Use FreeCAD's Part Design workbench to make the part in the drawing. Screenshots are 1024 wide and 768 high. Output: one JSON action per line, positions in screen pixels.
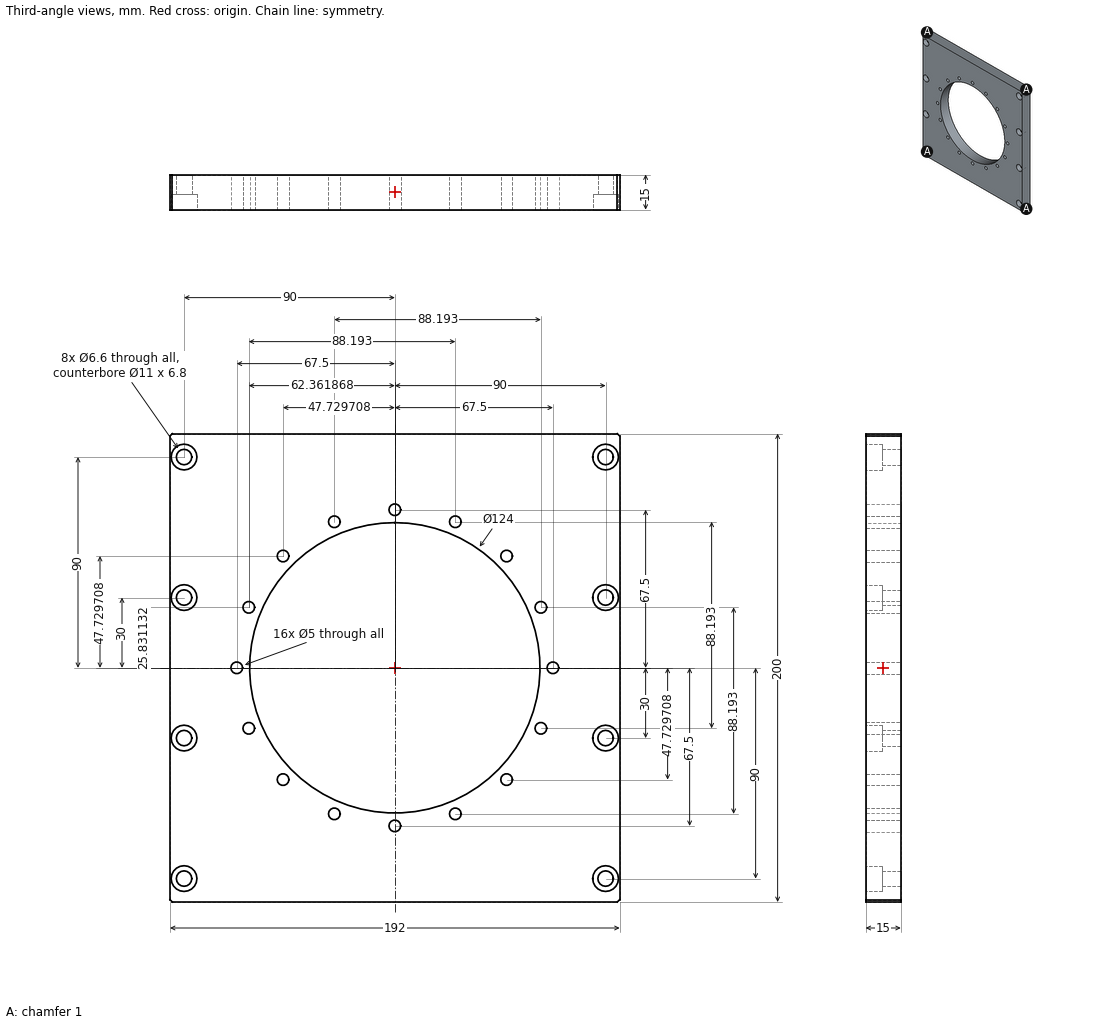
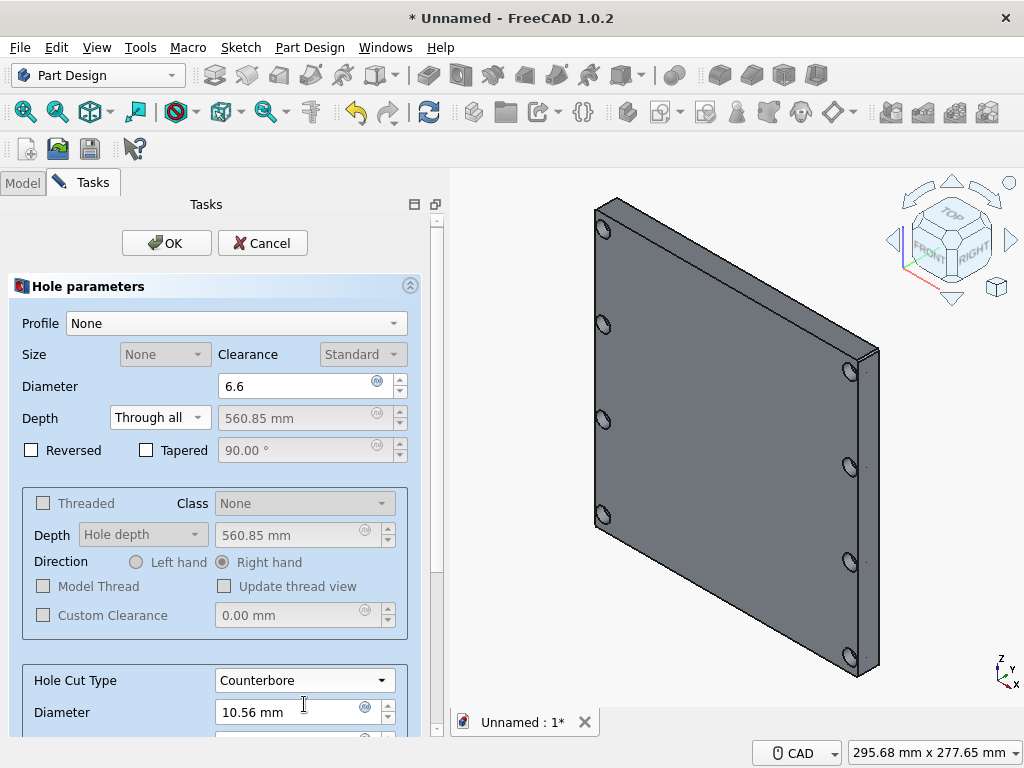
{"action": "triple_click", "coordinate": [298, 712]}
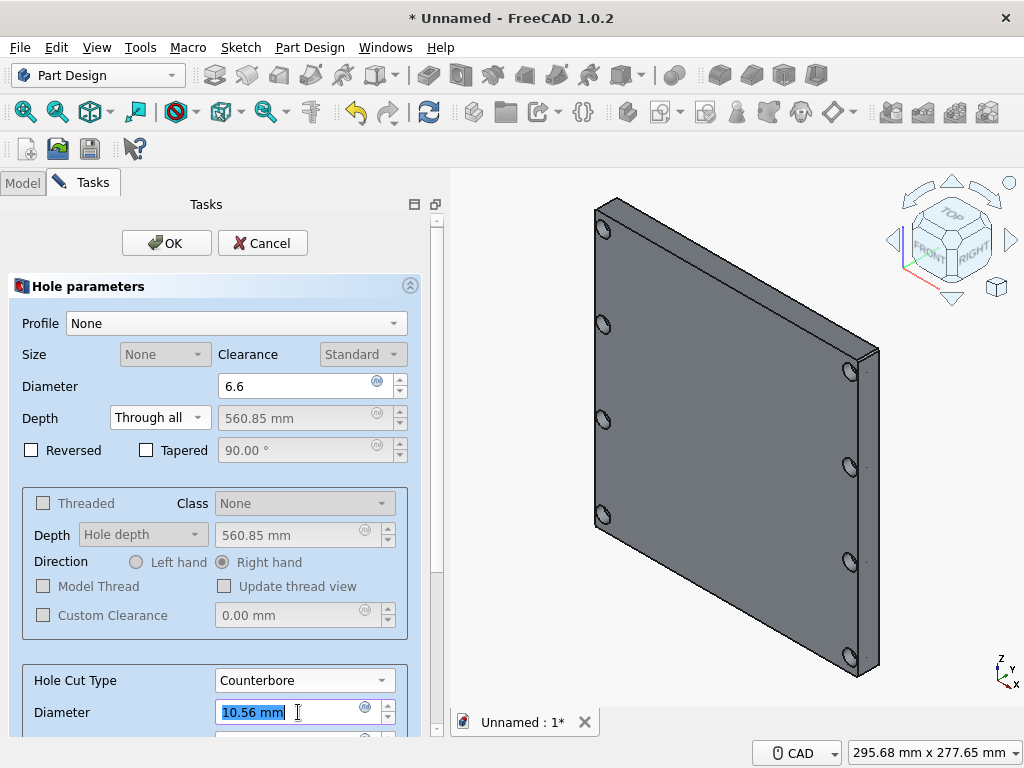
{"action": "type", "text": "11"}
{"action": "key", "text": "Tab"}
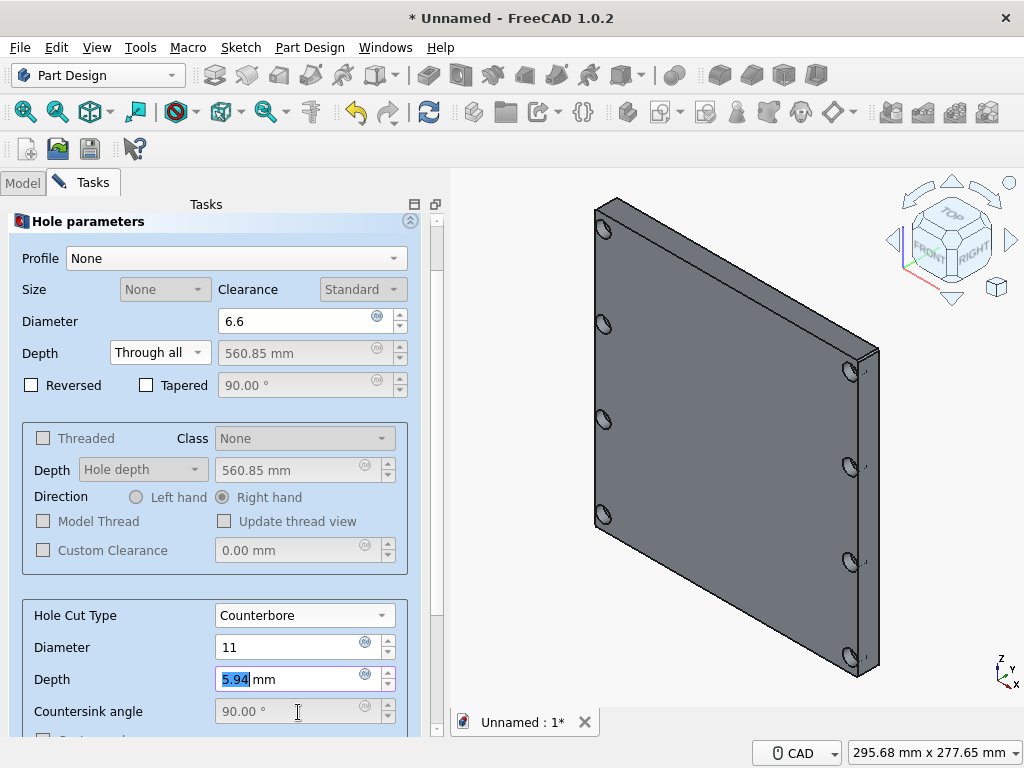
{"action": "type", "text": "6.8"}
{"action": "key", "text": "Tab"}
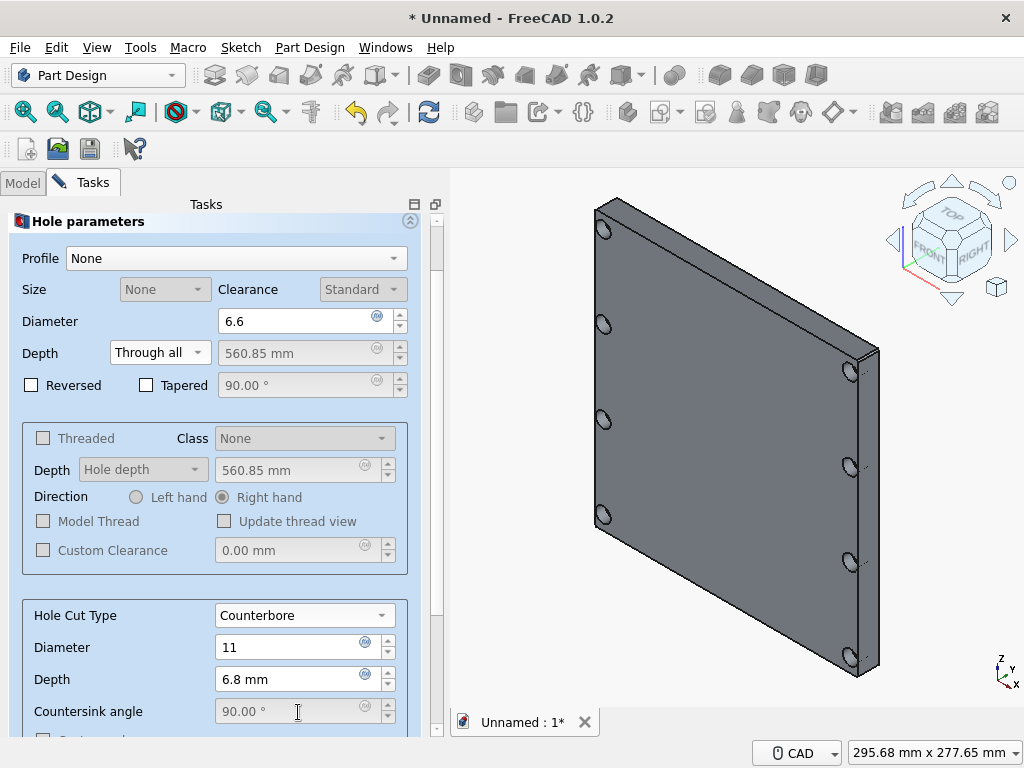
{"action": "scroll", "coordinate": [437, 475], "scroll_direction": "up", "scroll_amount": 2}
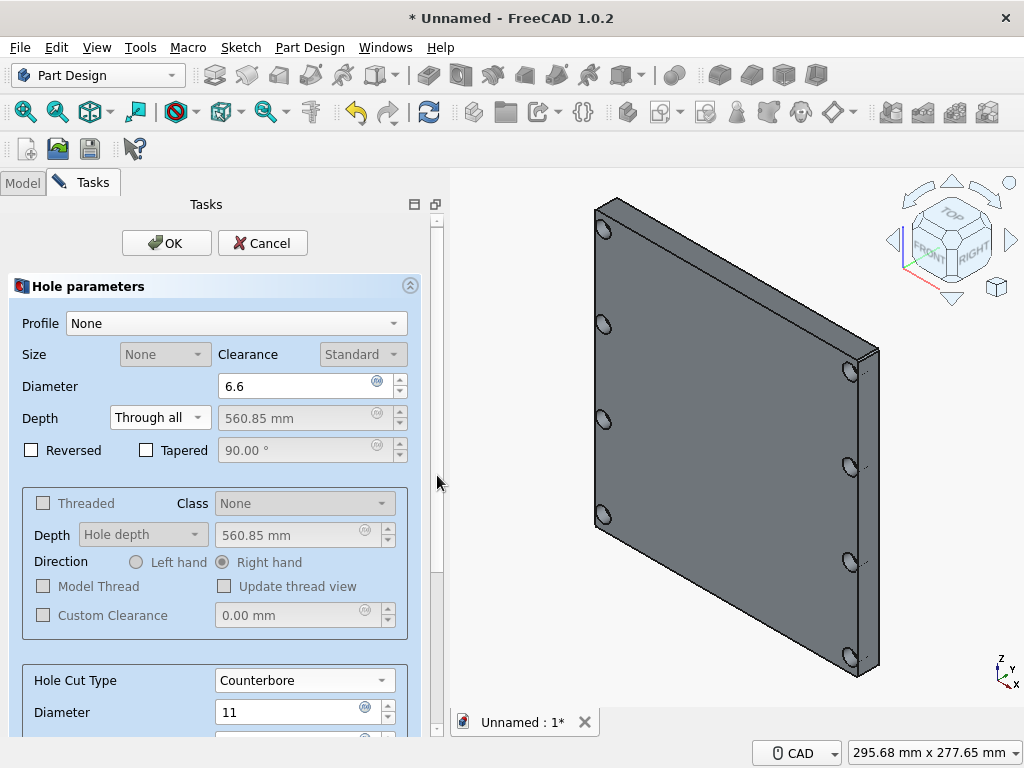
{"action": "left_click", "coordinate": [167, 243]}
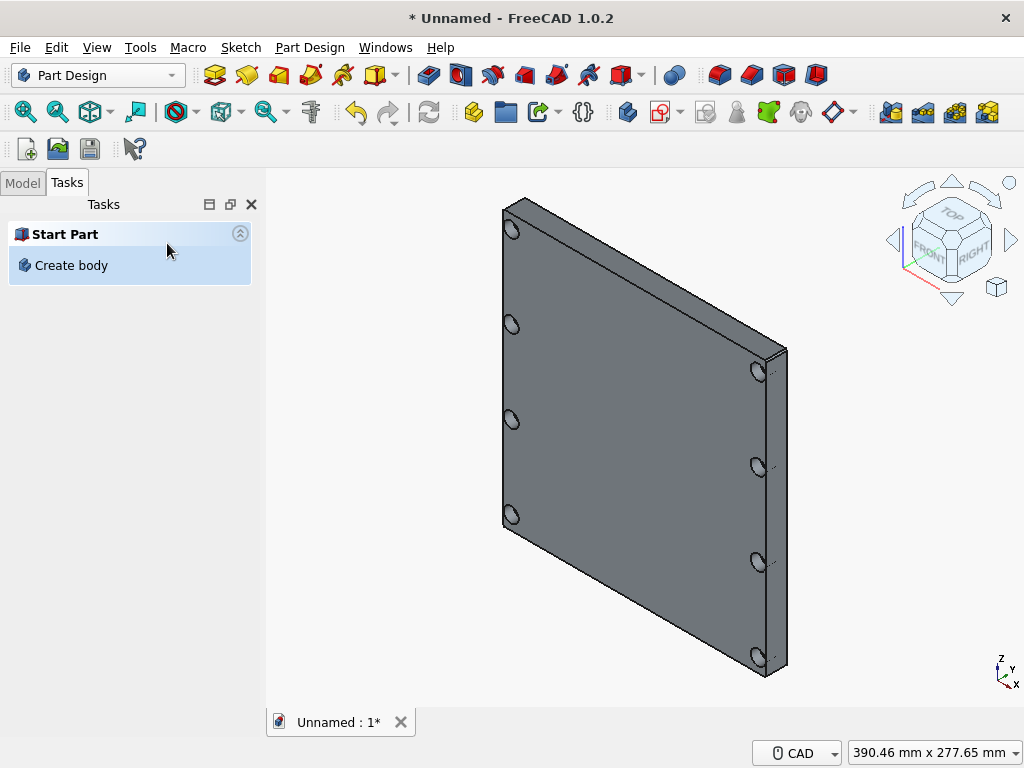
{"action": "key", "text": "4"}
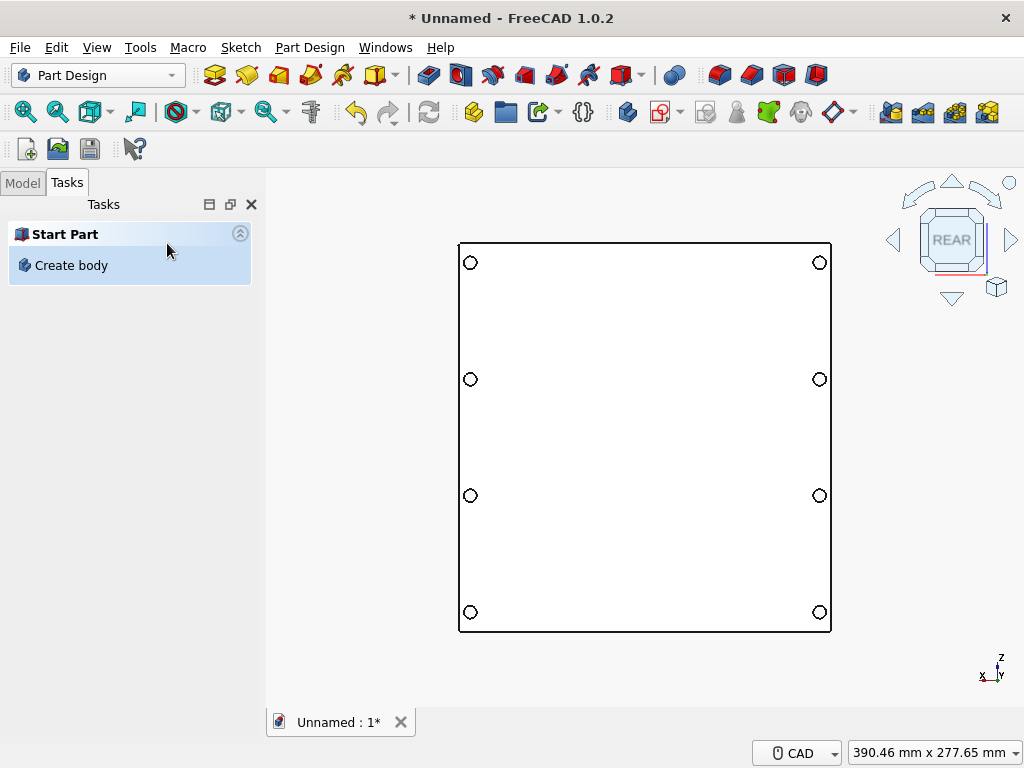
{"action": "left_click", "coordinate": [645, 436]}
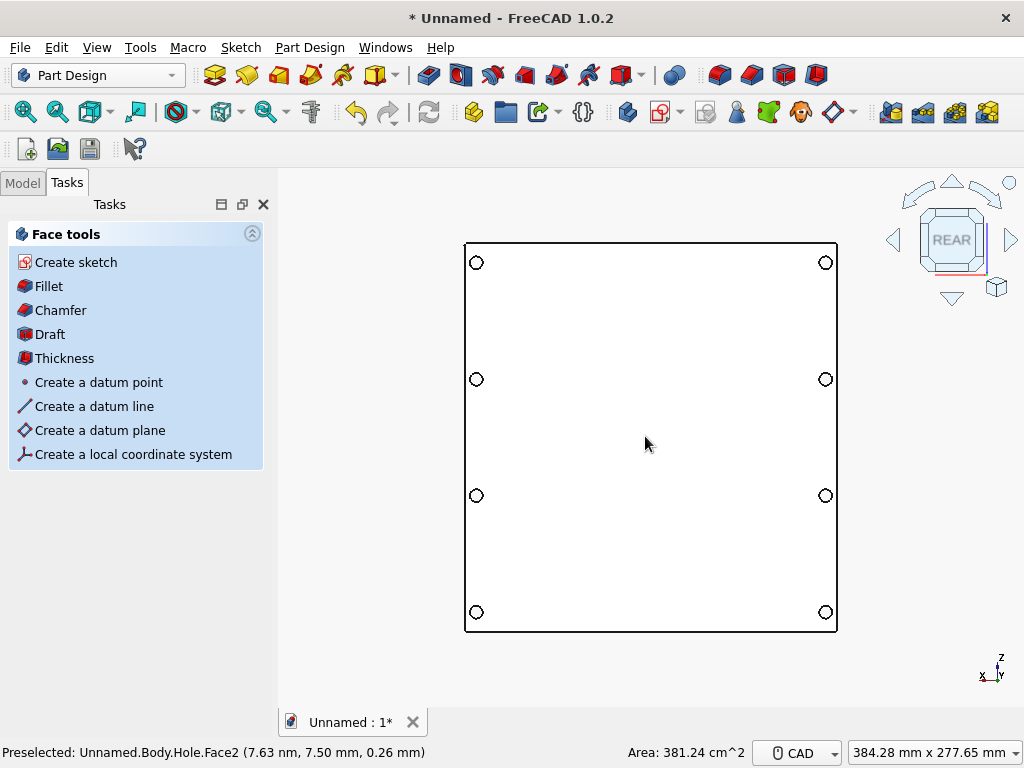
{"action": "left_click", "coordinate": [660, 112]}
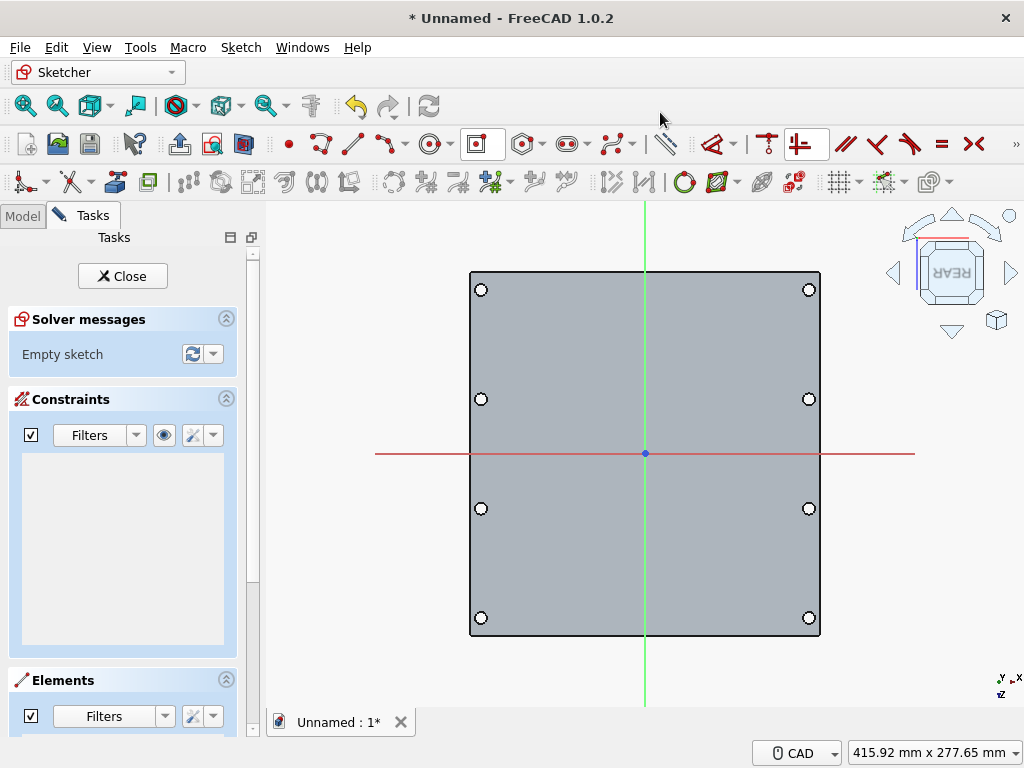
{"action": "scroll", "coordinate": [784, 454], "scroll_direction": "up", "scroll_amount": 2}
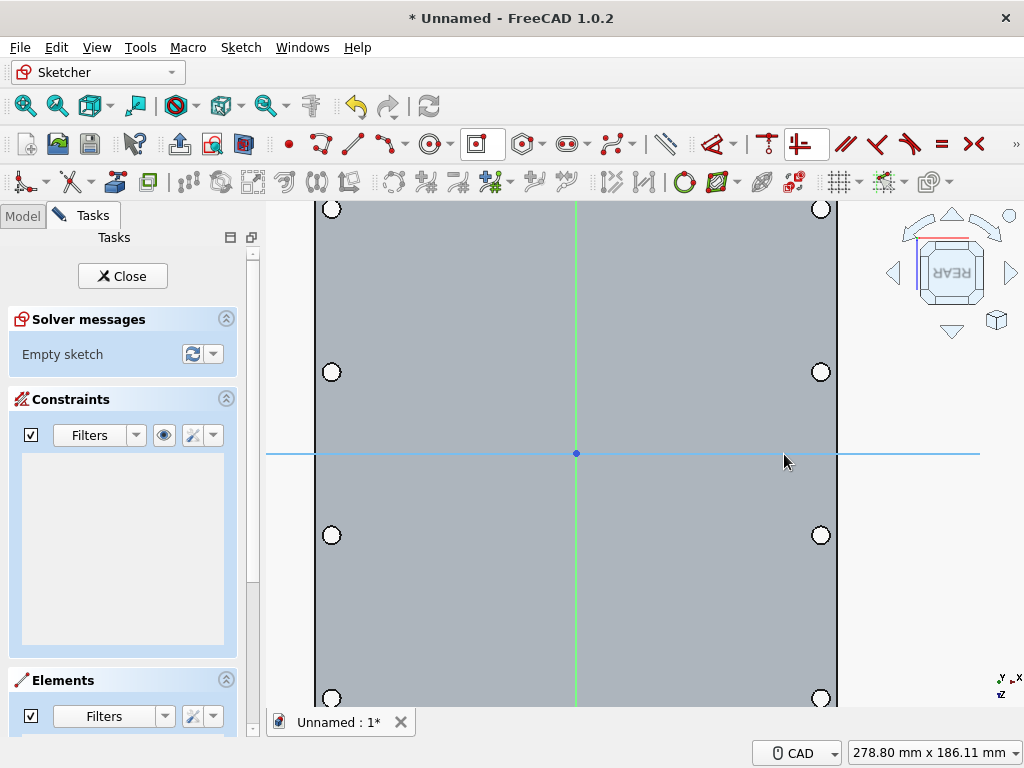
{"action": "left_click", "coordinate": [430, 144]}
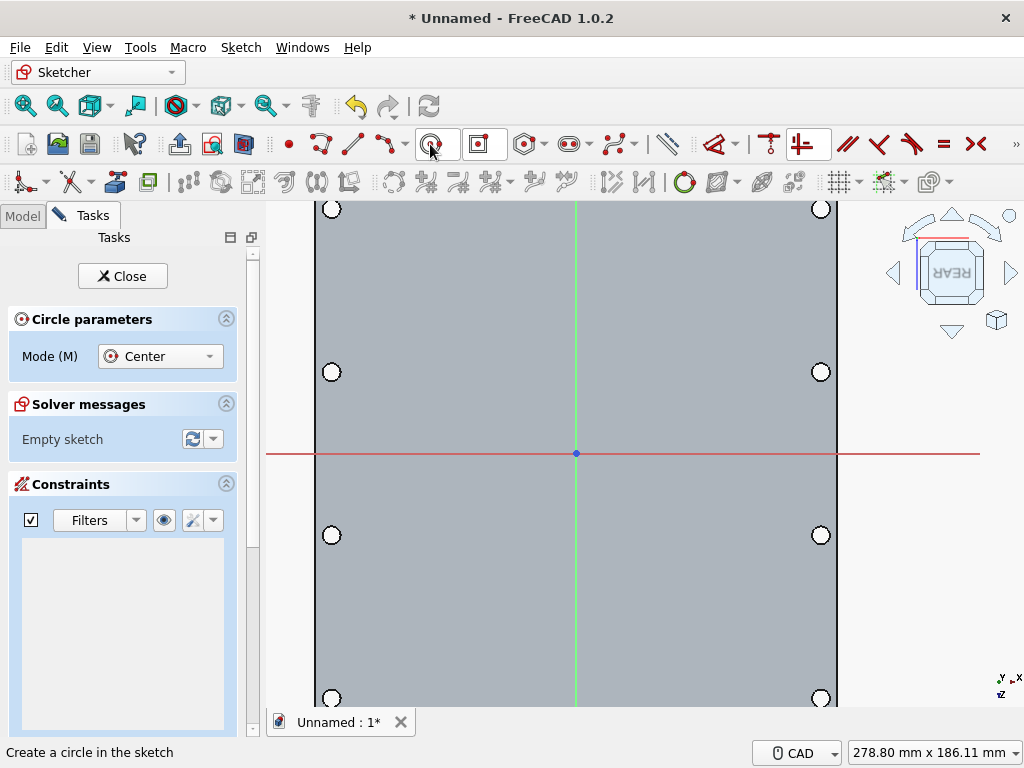
{"action": "left_click", "coordinate": [576, 454]}
{"action": "mouse_move", "coordinate": [695, 335]}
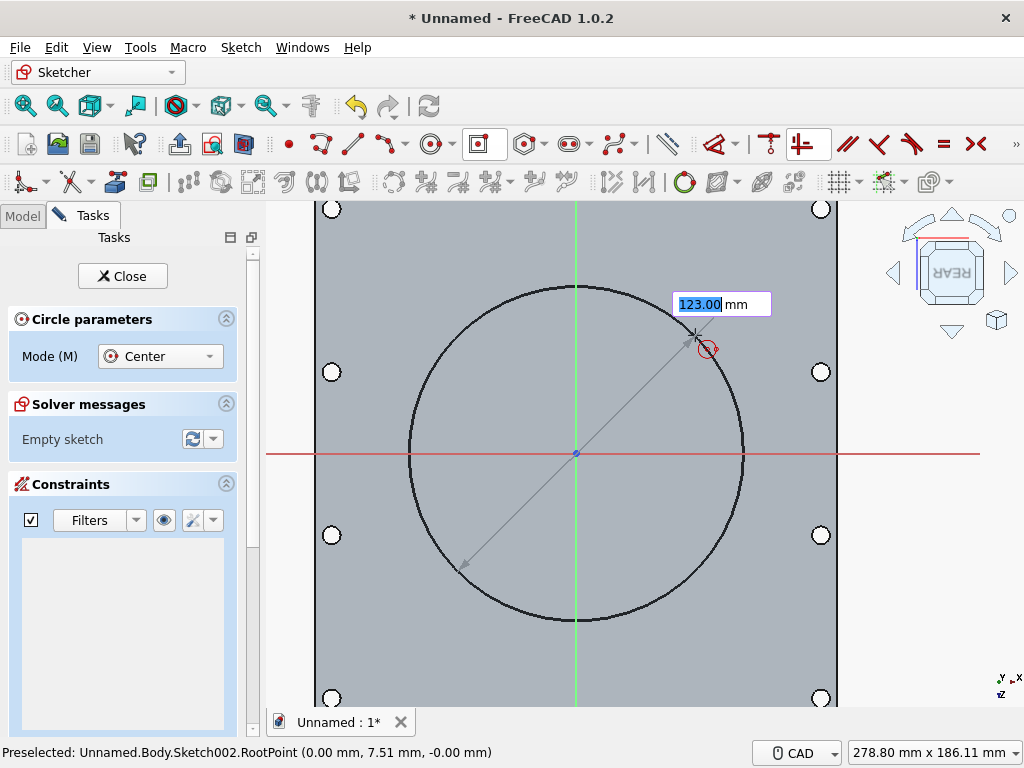
{"action": "type", "text": "124"}
{"action": "key", "text": "Return"}
{"action": "key", "text": "Escape"}